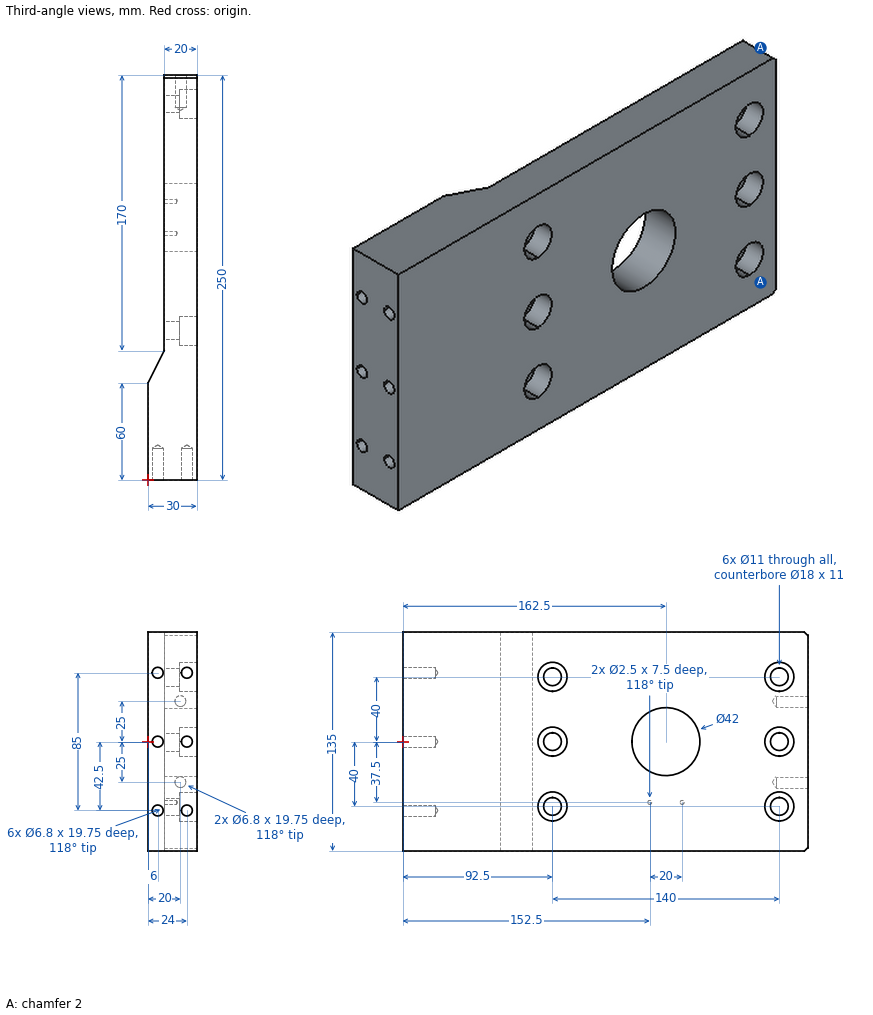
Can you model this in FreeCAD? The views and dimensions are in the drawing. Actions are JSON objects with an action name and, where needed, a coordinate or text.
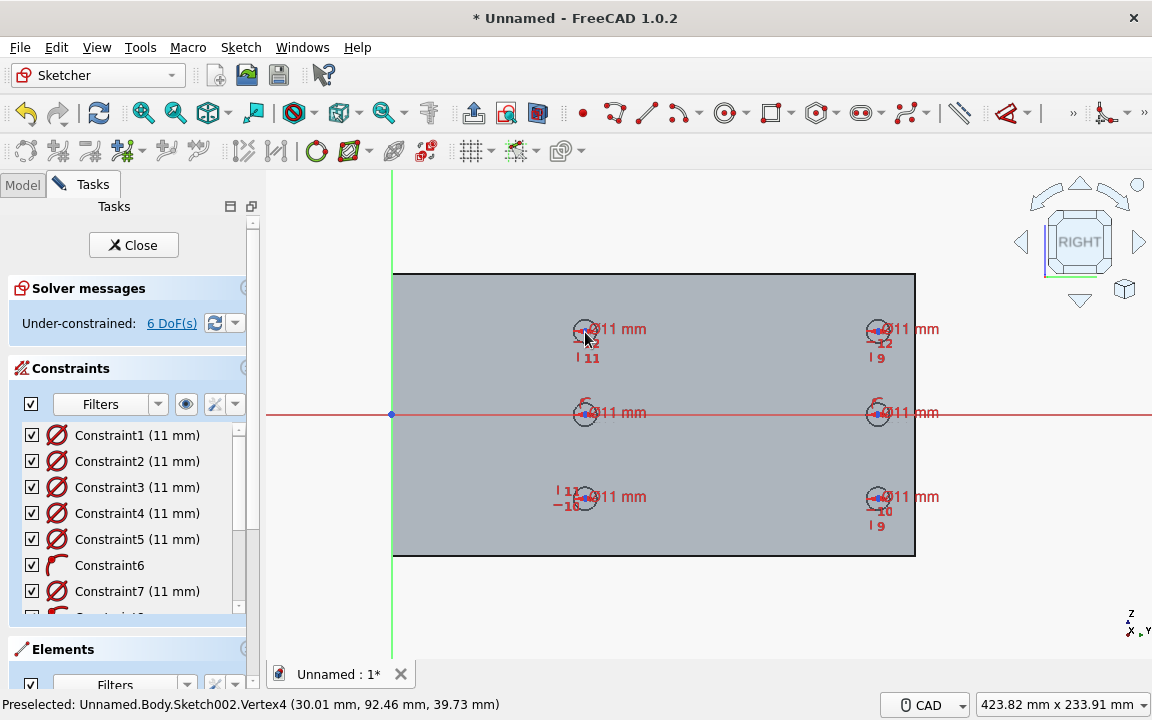
{"action": "left_click", "coordinate": [878, 331]}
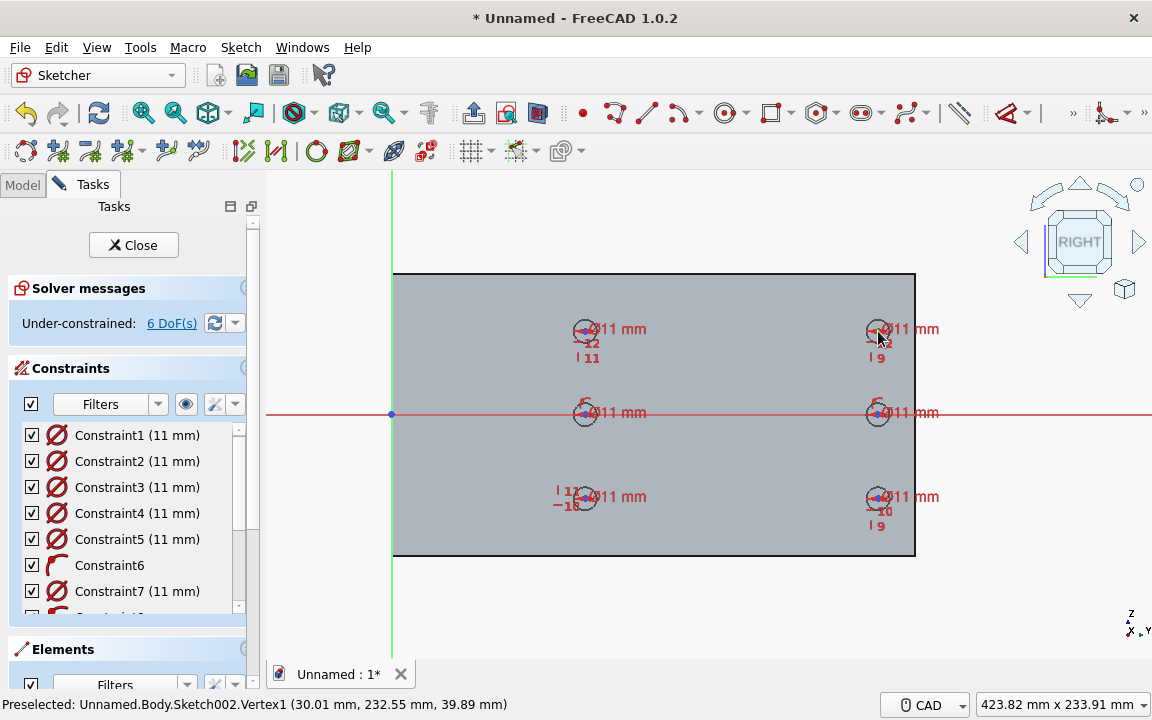
{"action": "left_click", "coordinate": [878, 415]}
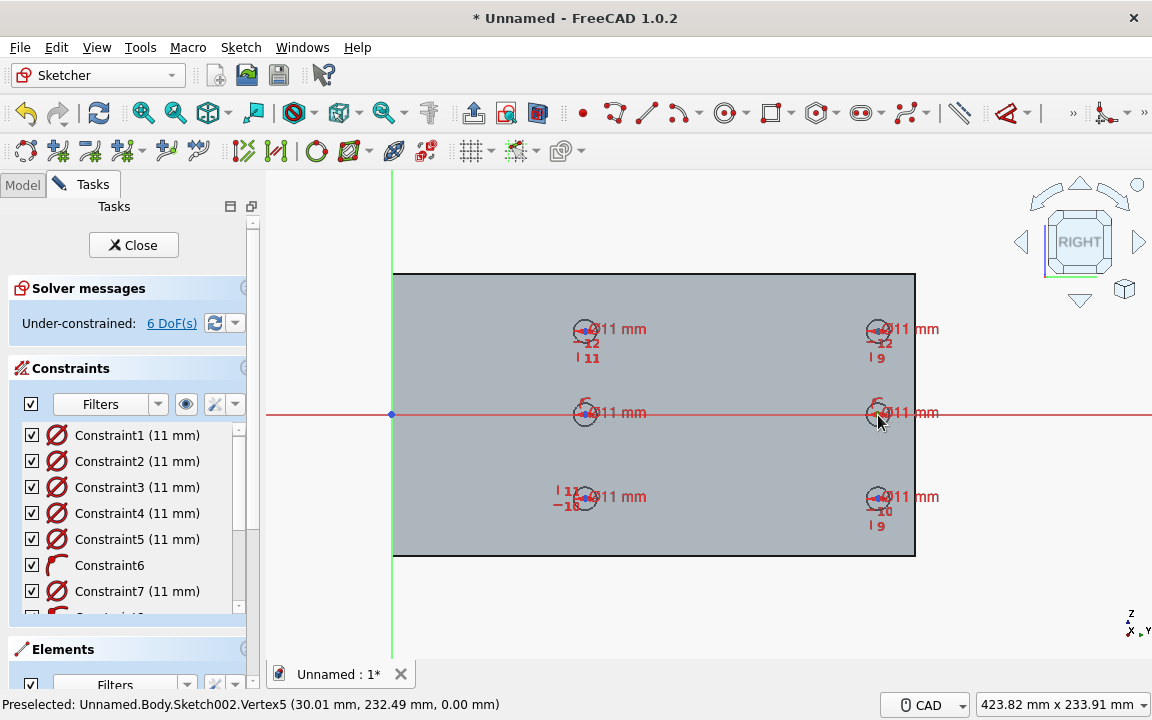
{"action": "key", "text": "v"}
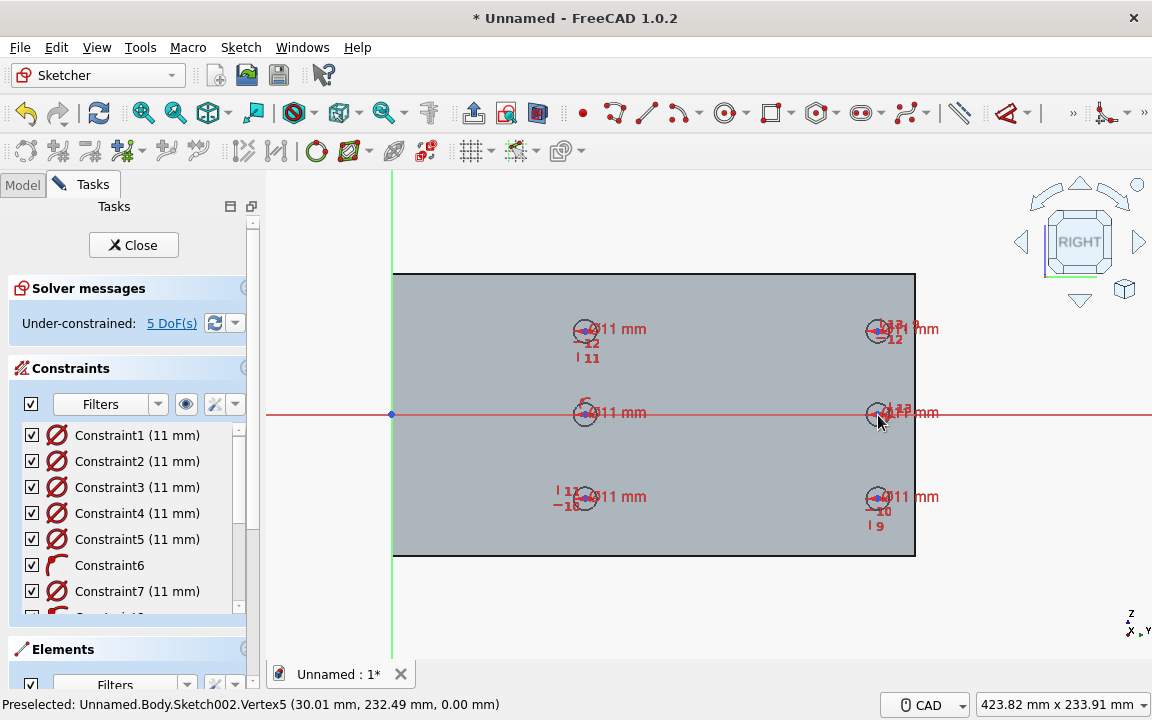
{"action": "left_click", "coordinate": [585, 499]}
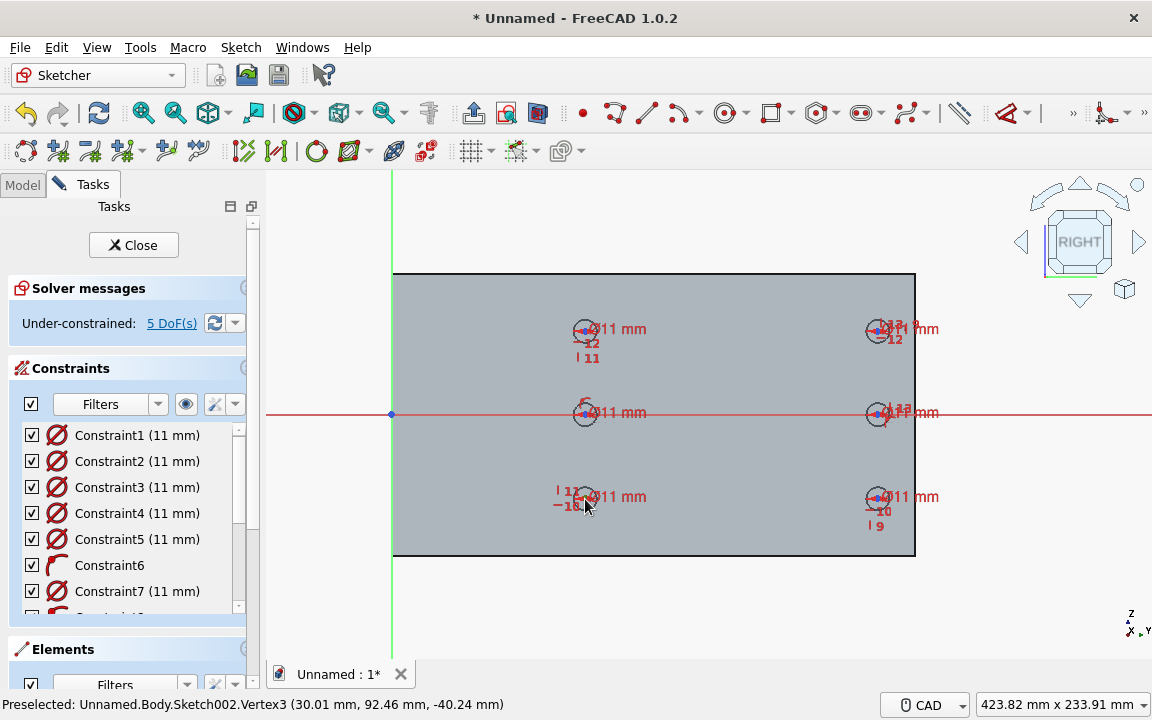
{"action": "left_click", "coordinate": [585, 415]}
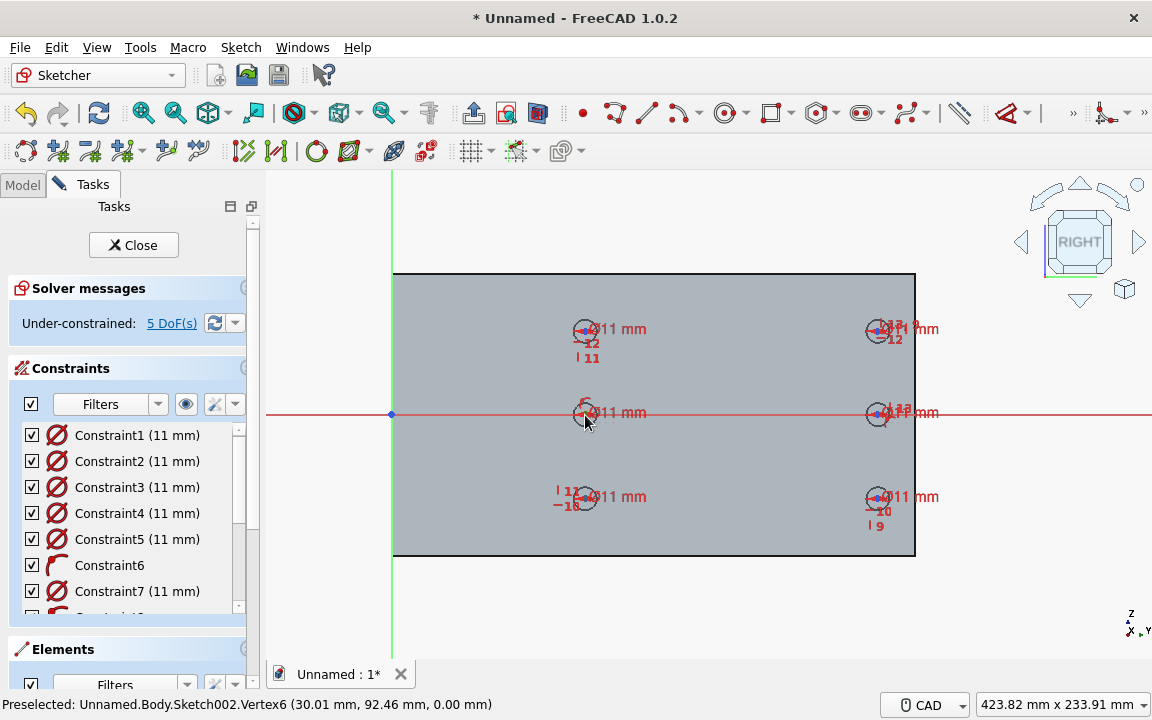
{"action": "key", "text": "v"}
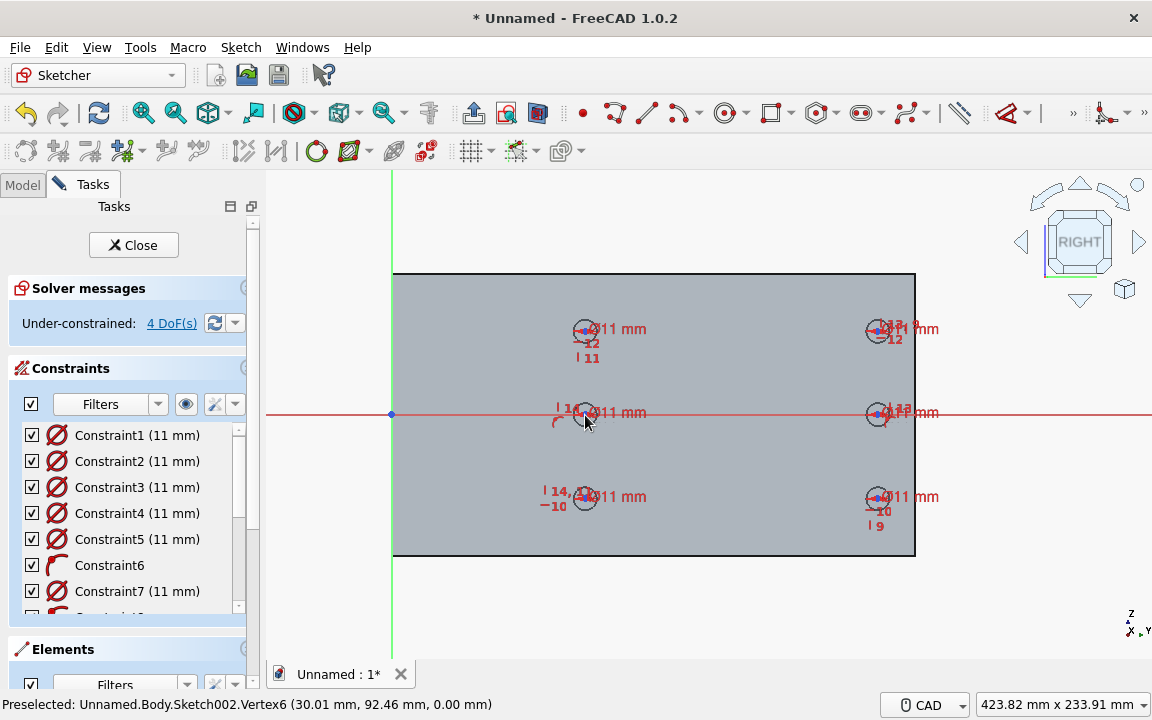
{"action": "left_click", "coordinate": [1006, 114]}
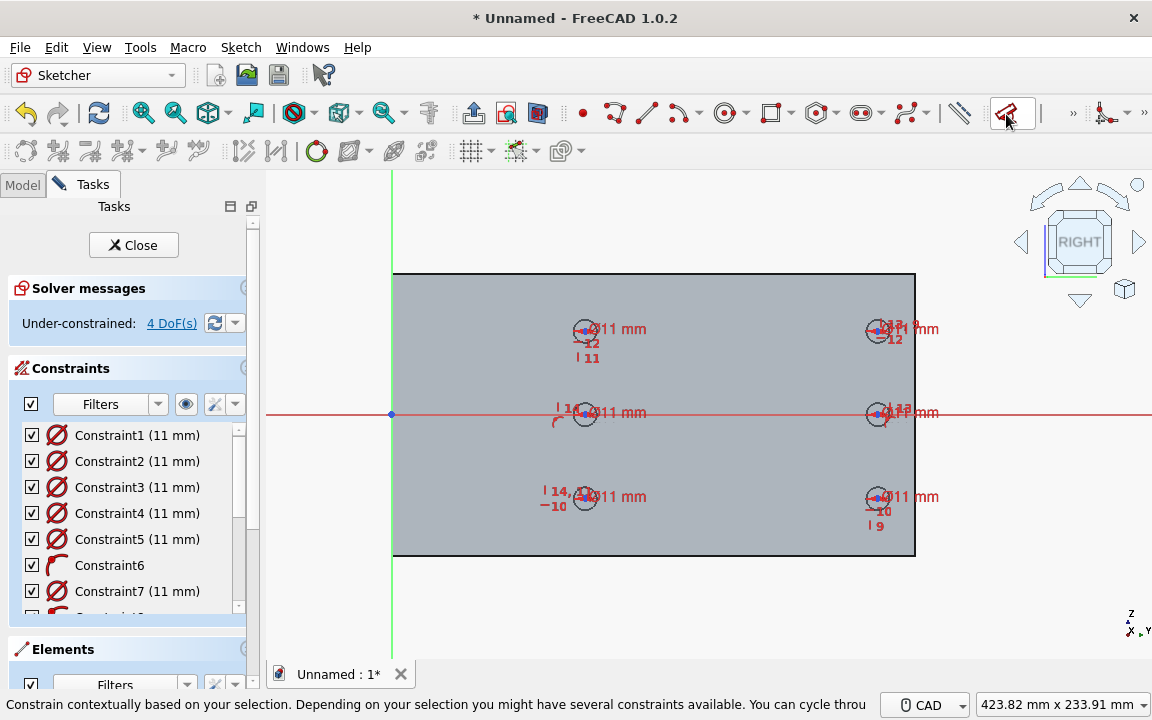
{"action": "left_click", "coordinate": [878, 331]}
{"action": "left_click", "coordinate": [358, 373]}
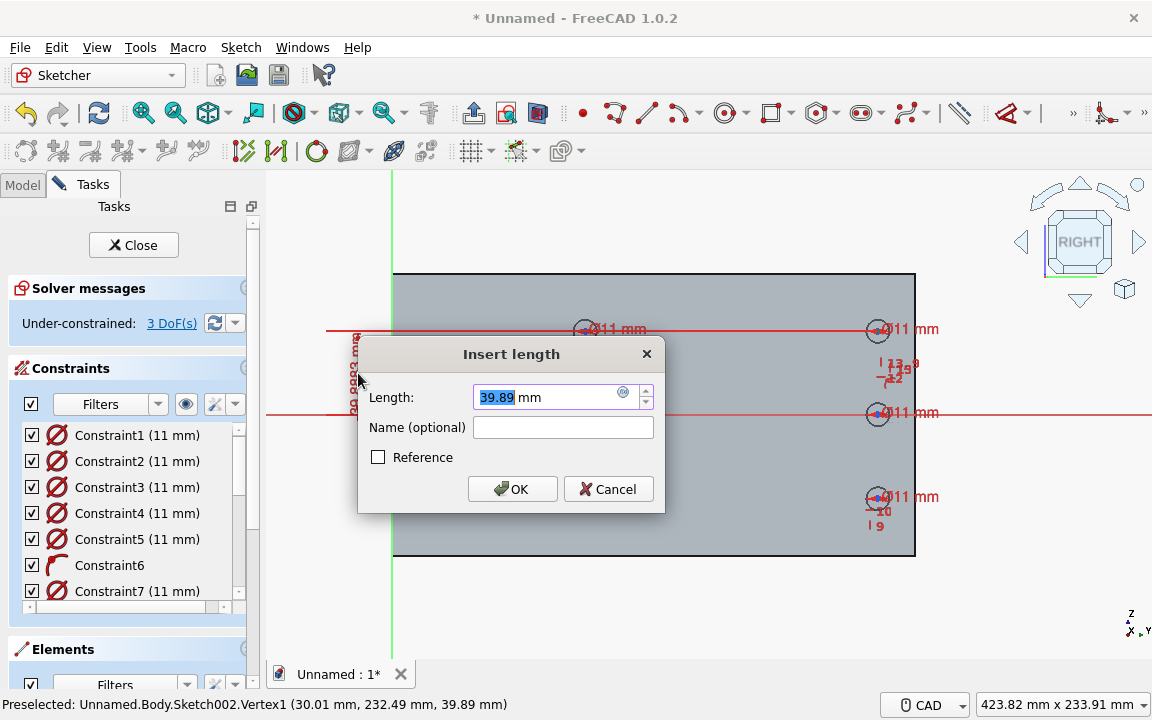
{"action": "type", "text": "40"}
{"action": "key", "text": "Return"}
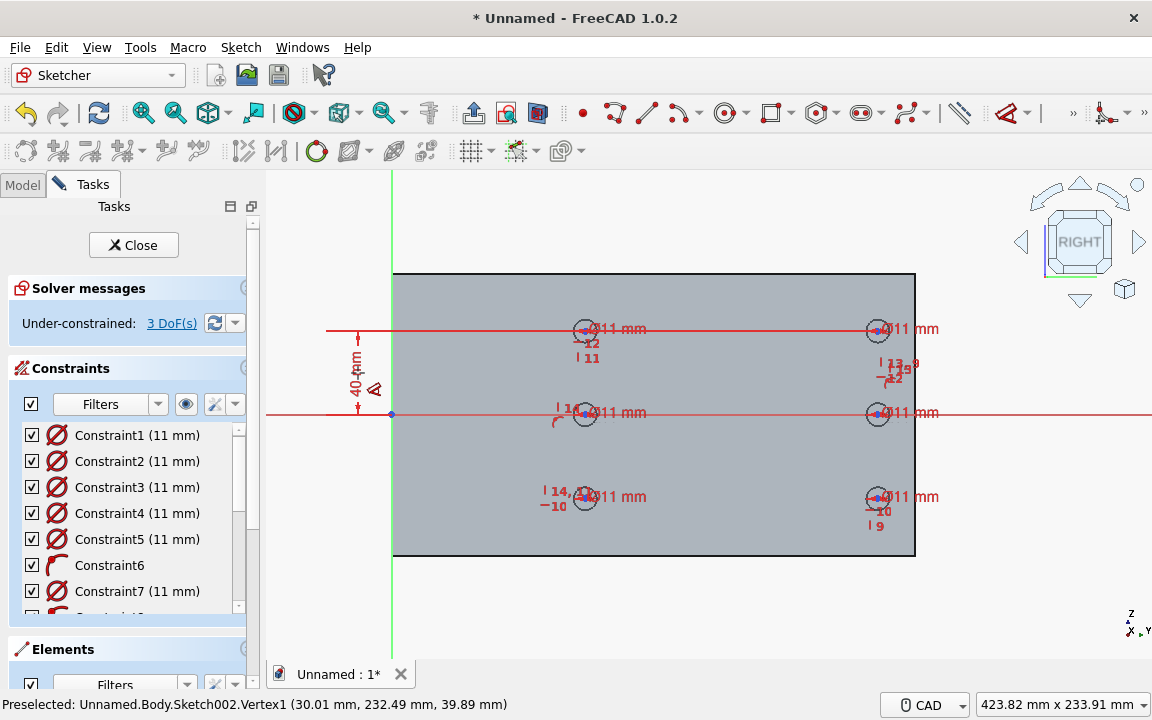
{"action": "left_click", "coordinate": [878, 499]}
{"action": "left_click", "coordinate": [358, 457]}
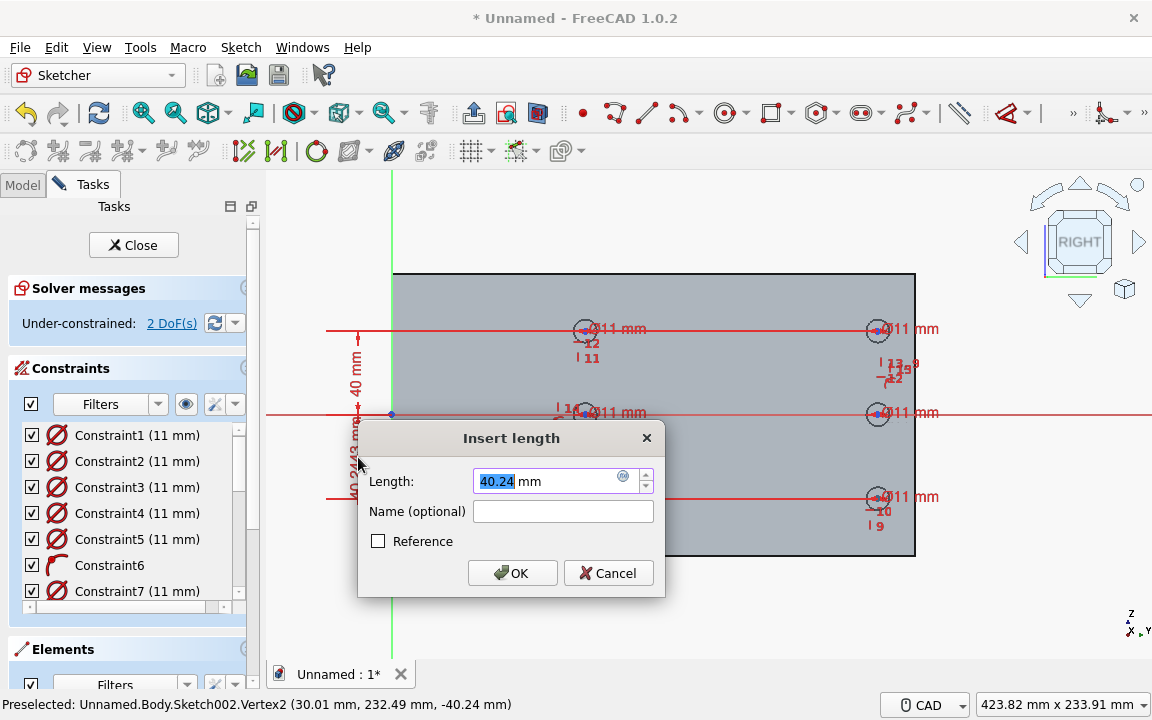
{"action": "type", "text": "40"}
{"action": "key", "text": "Return"}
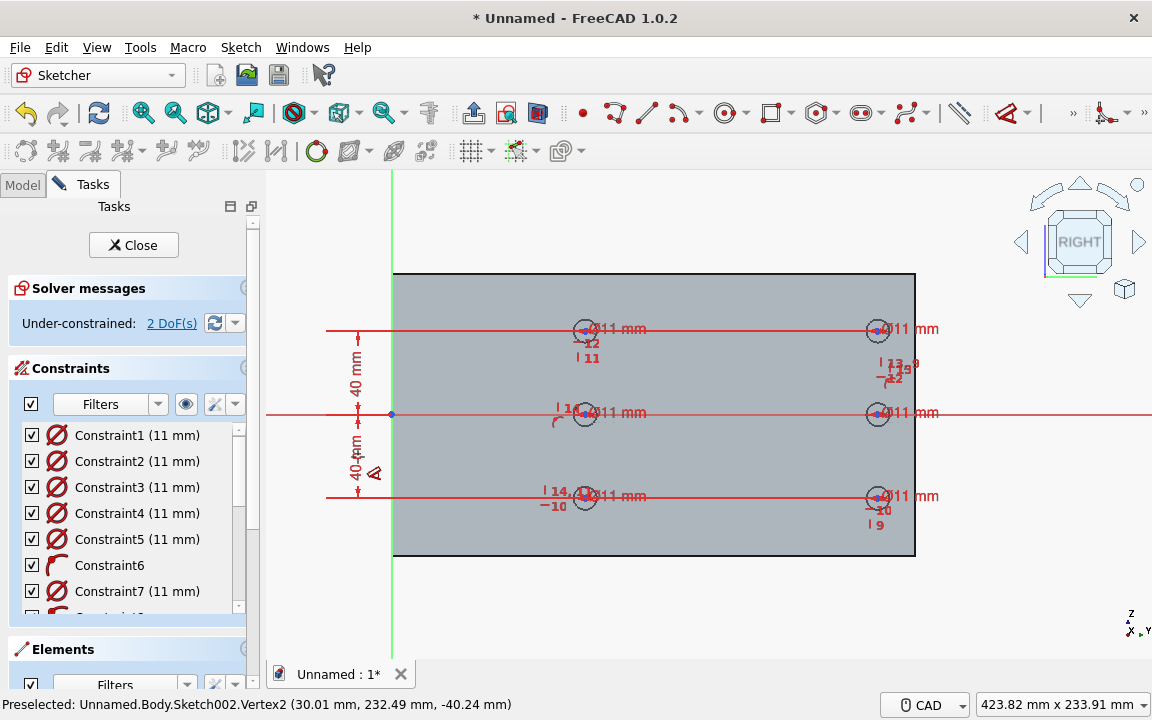
{"action": "left_click", "coordinate": [585, 498]}
{"action": "left_click", "coordinate": [489, 532]}